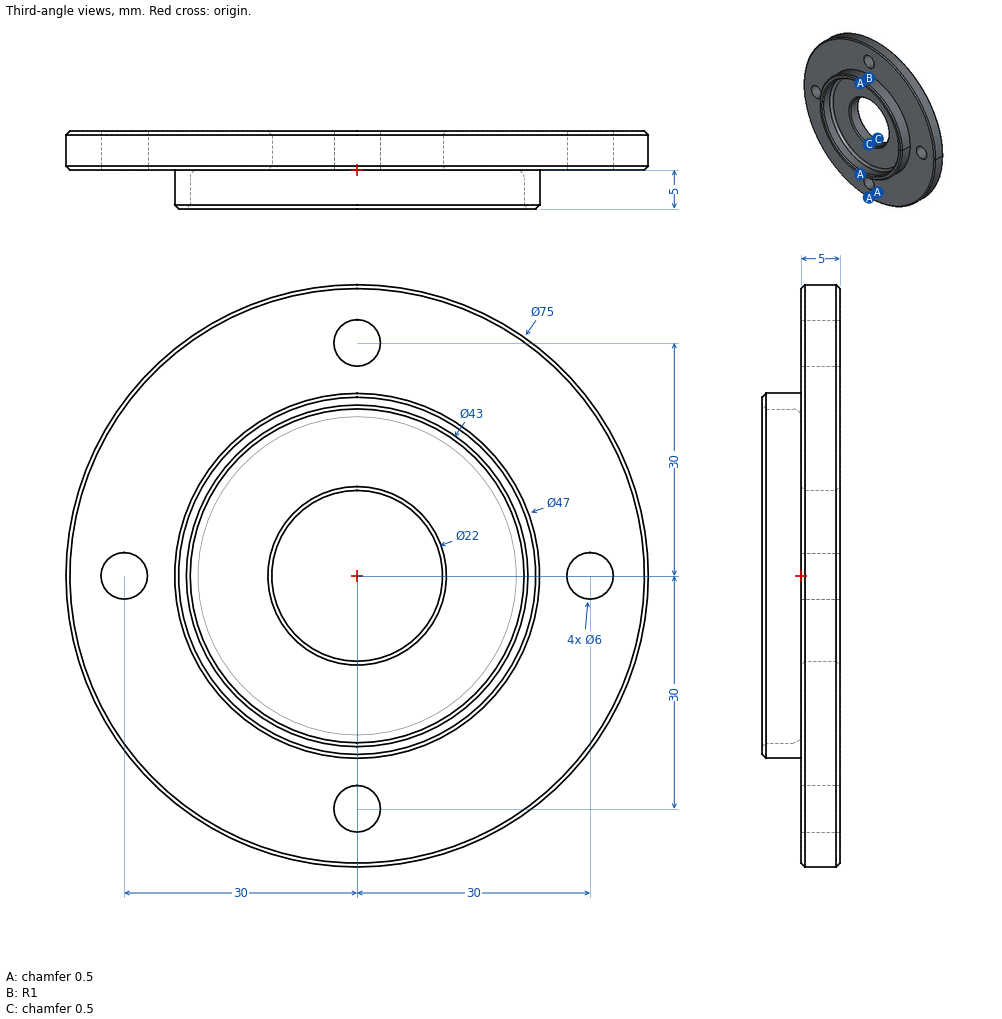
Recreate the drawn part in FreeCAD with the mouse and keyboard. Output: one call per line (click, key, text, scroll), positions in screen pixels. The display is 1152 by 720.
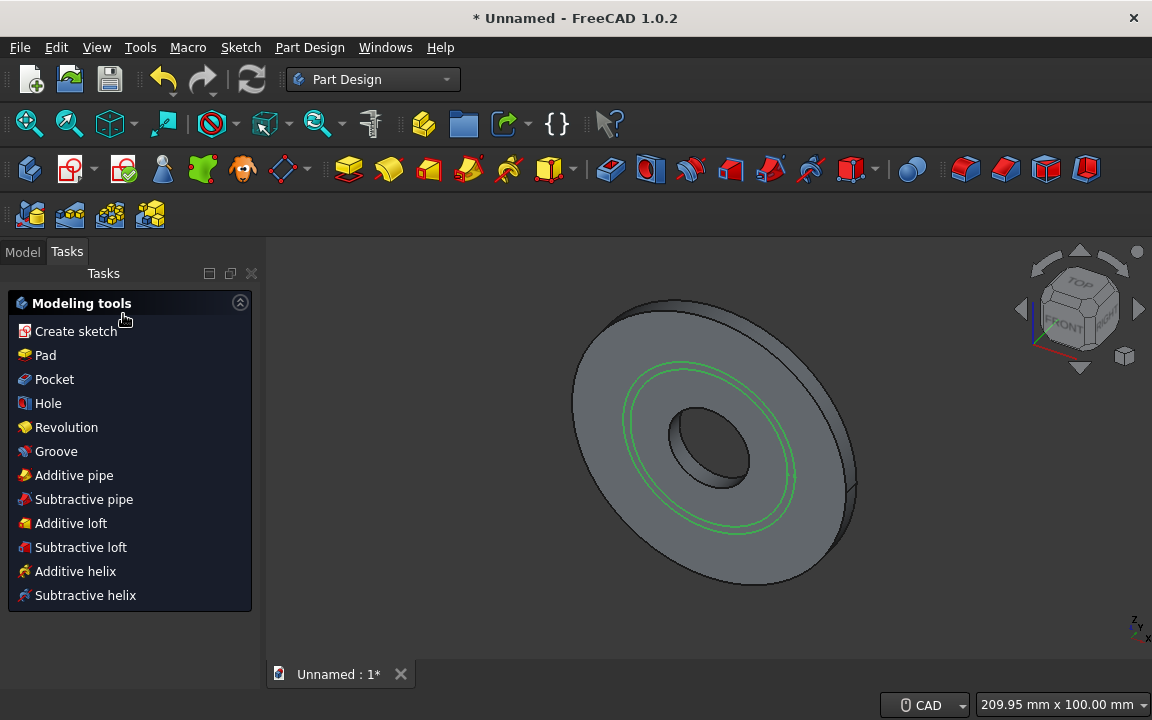
click(350, 170)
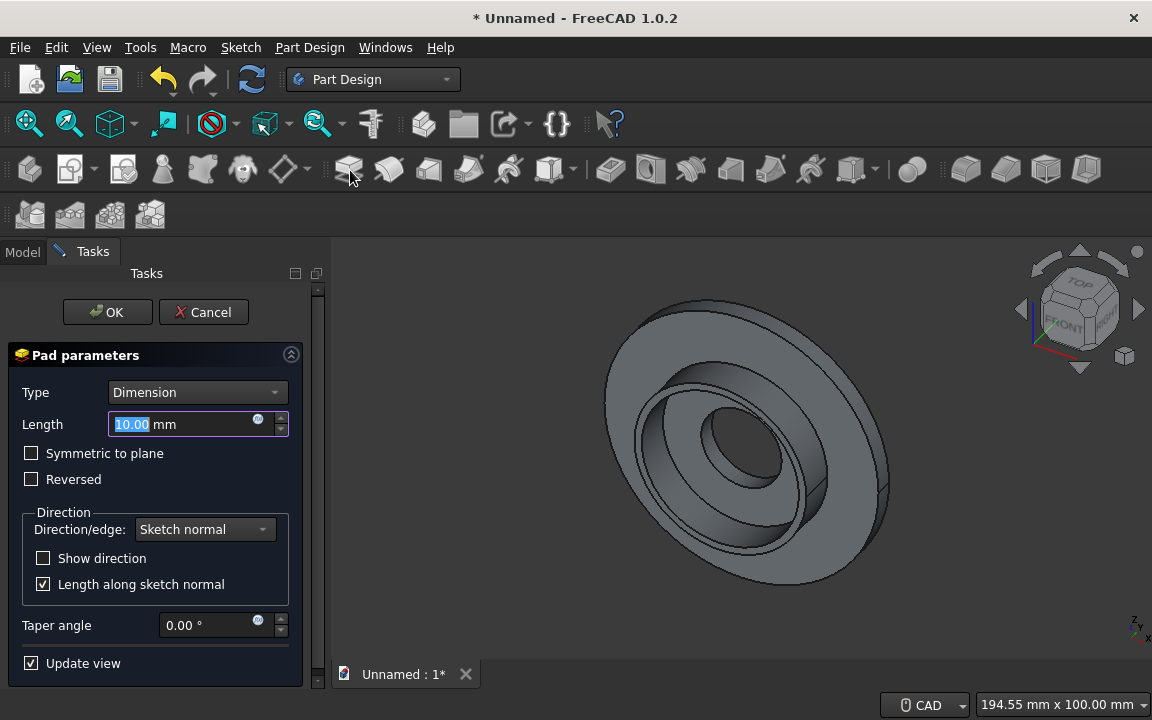
text(5)
key(Tab)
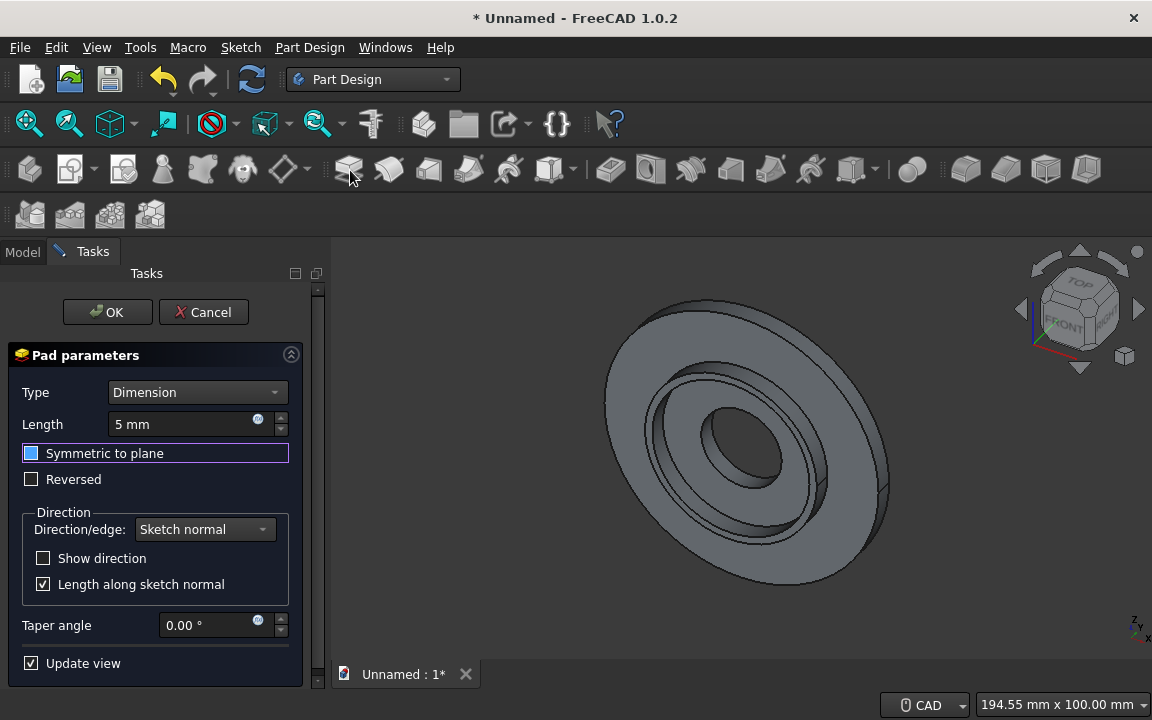
click(108, 312)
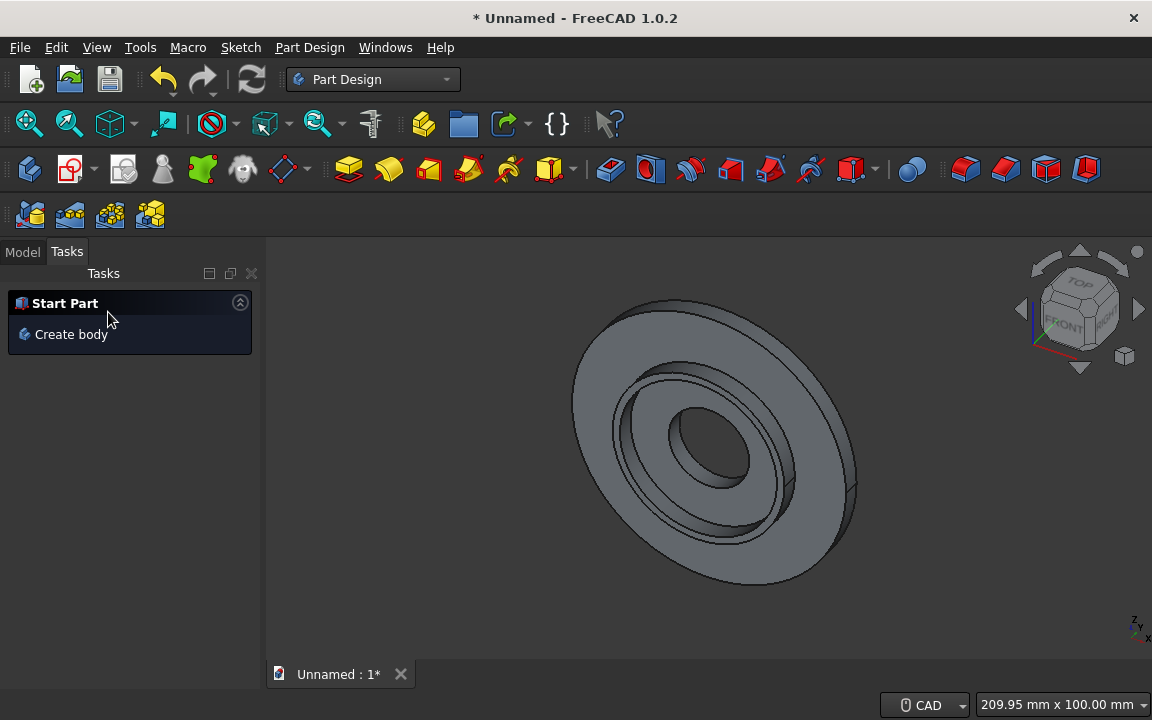
key(4)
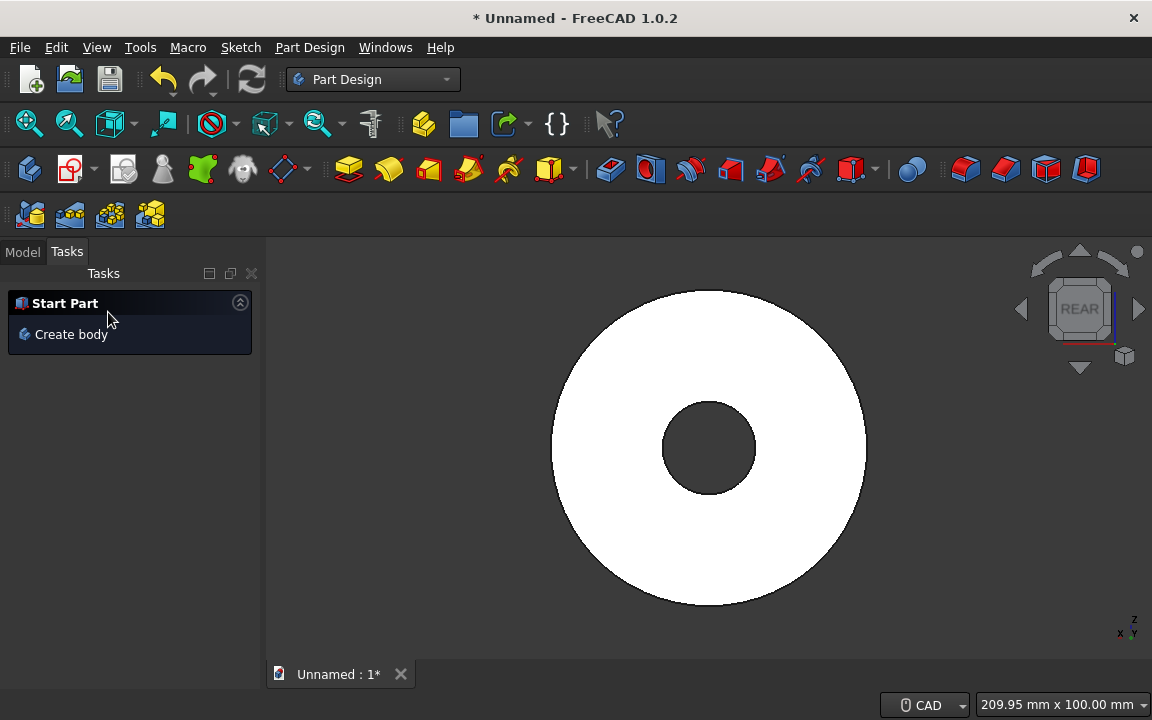
click(754, 357)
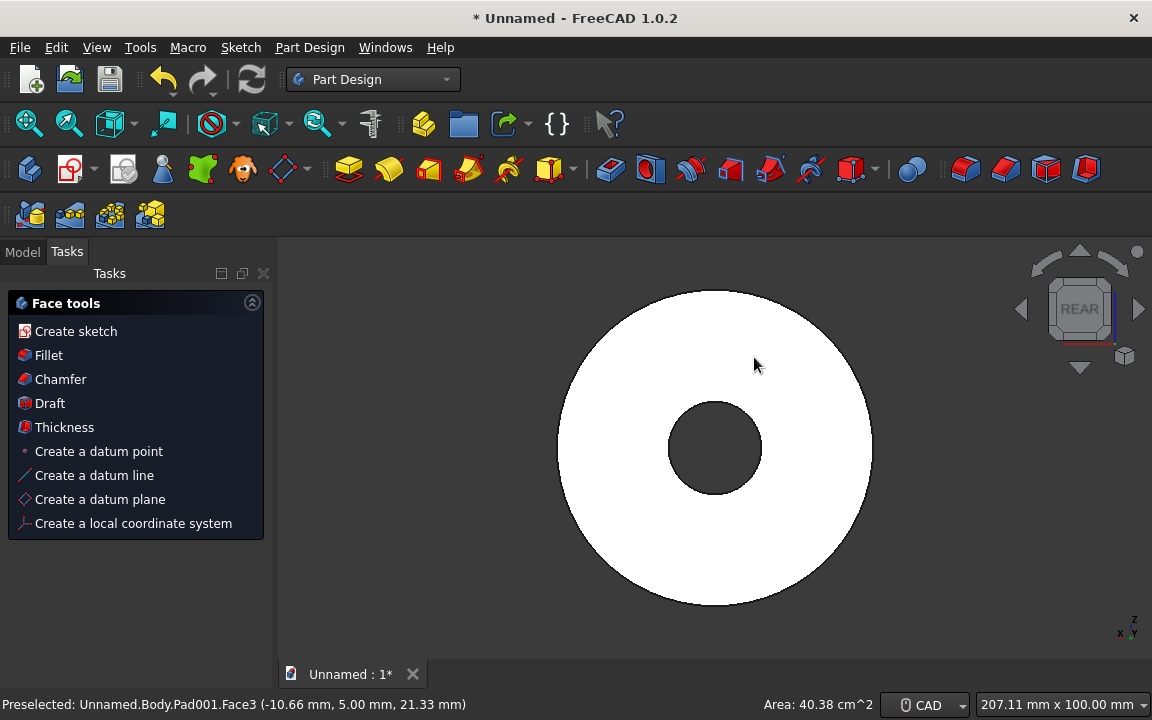
click(70, 170)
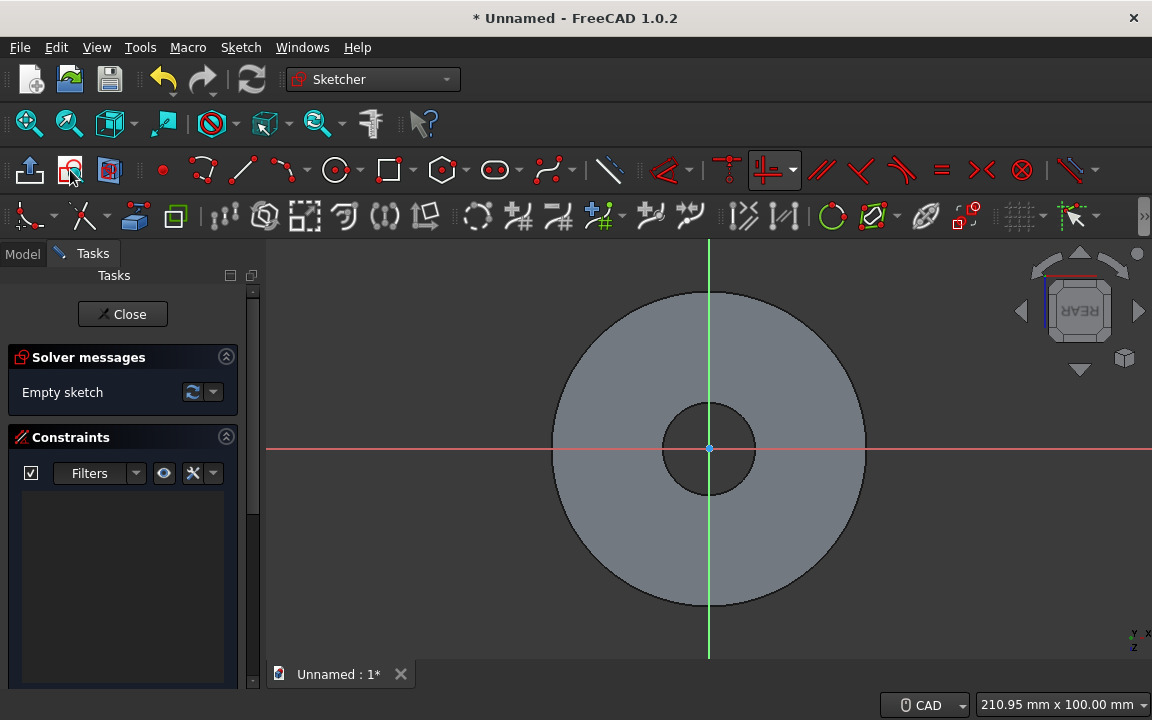
key(g)
key(c)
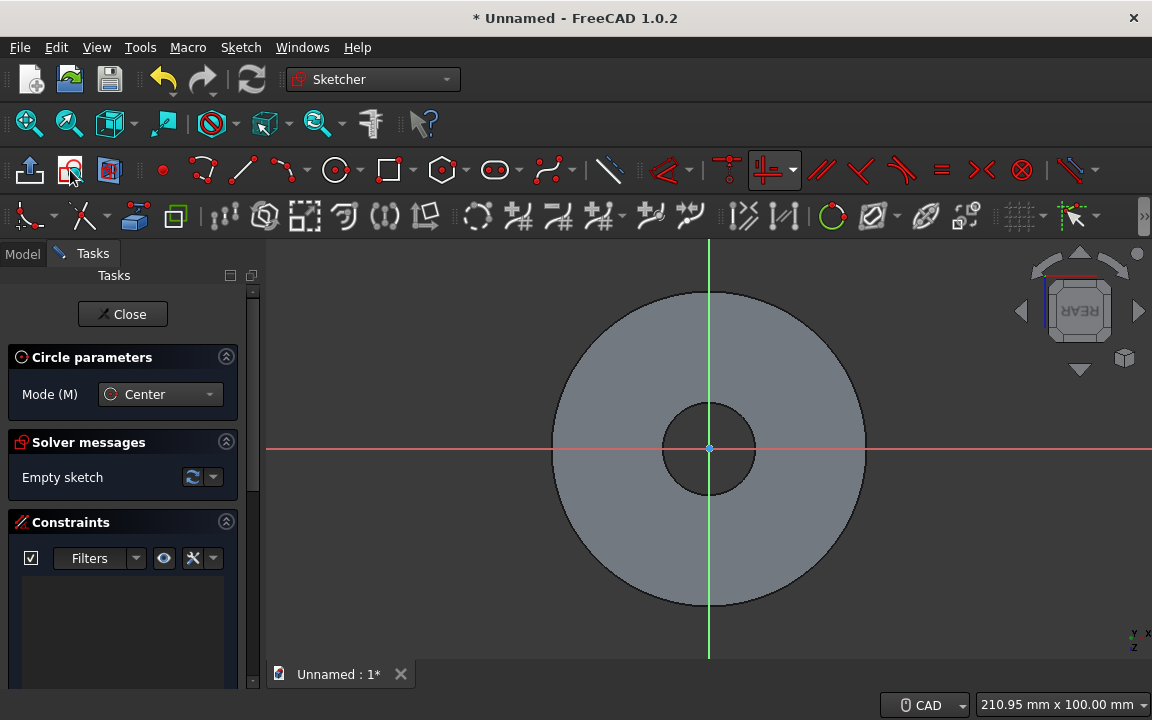
scroll(835, 449, up, 3)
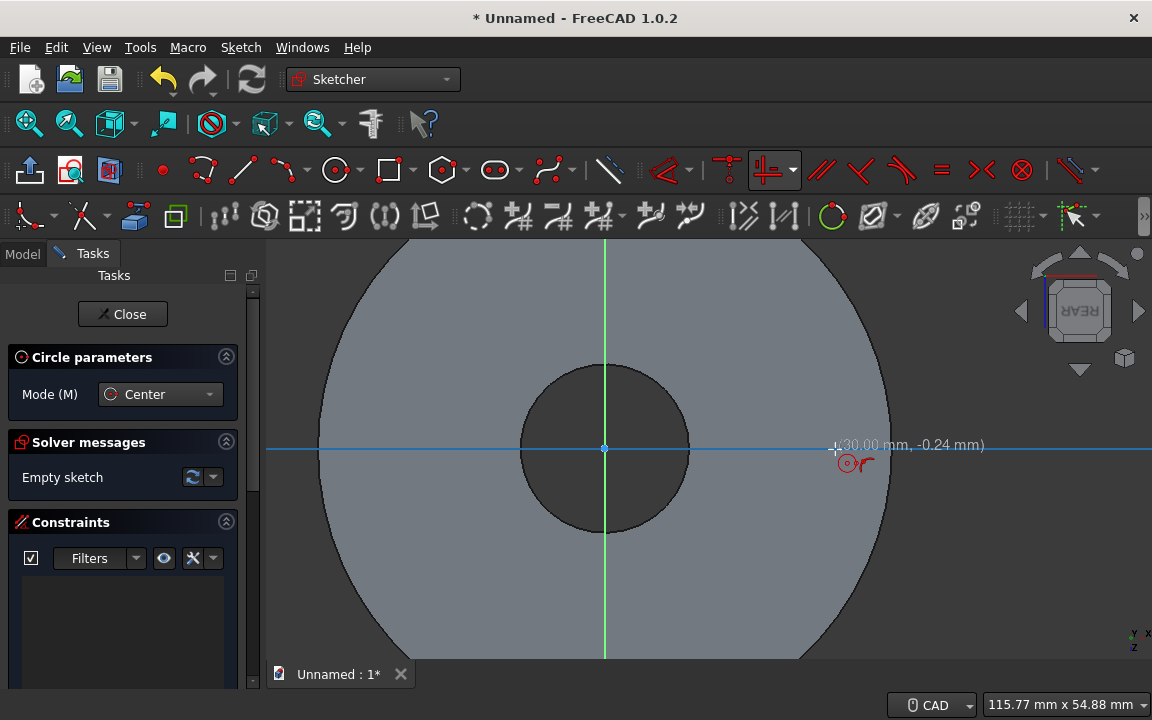
click(834, 449)
move(851, 432)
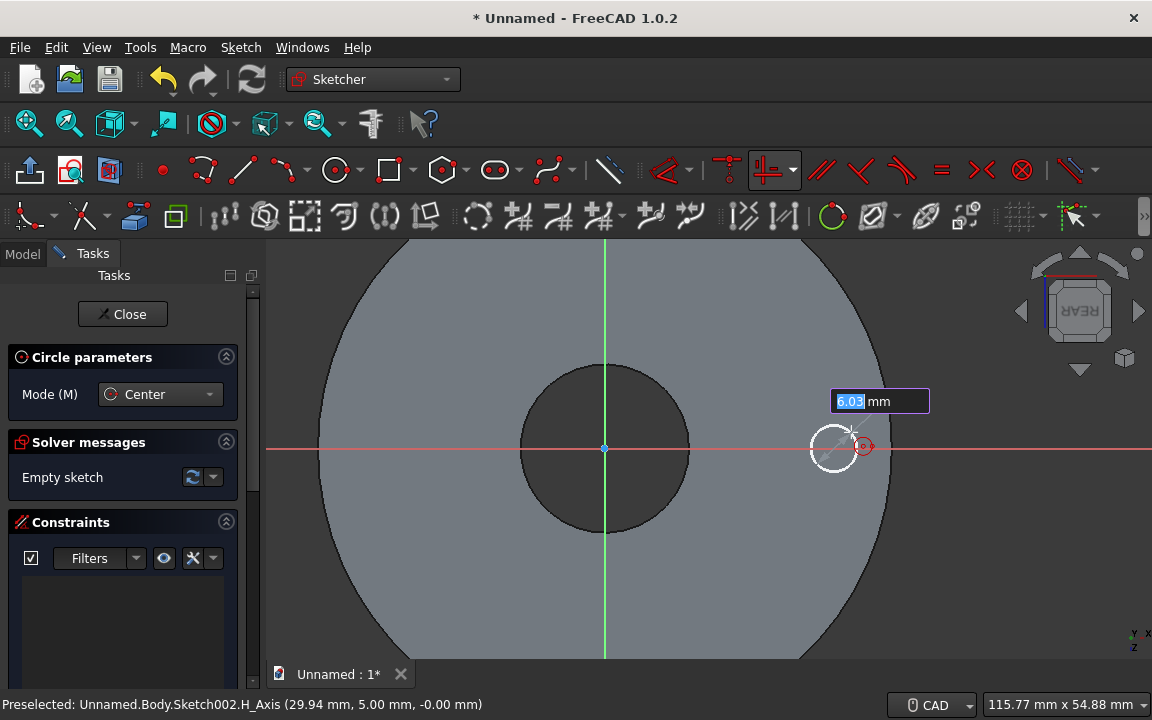
text(6)
key(Return)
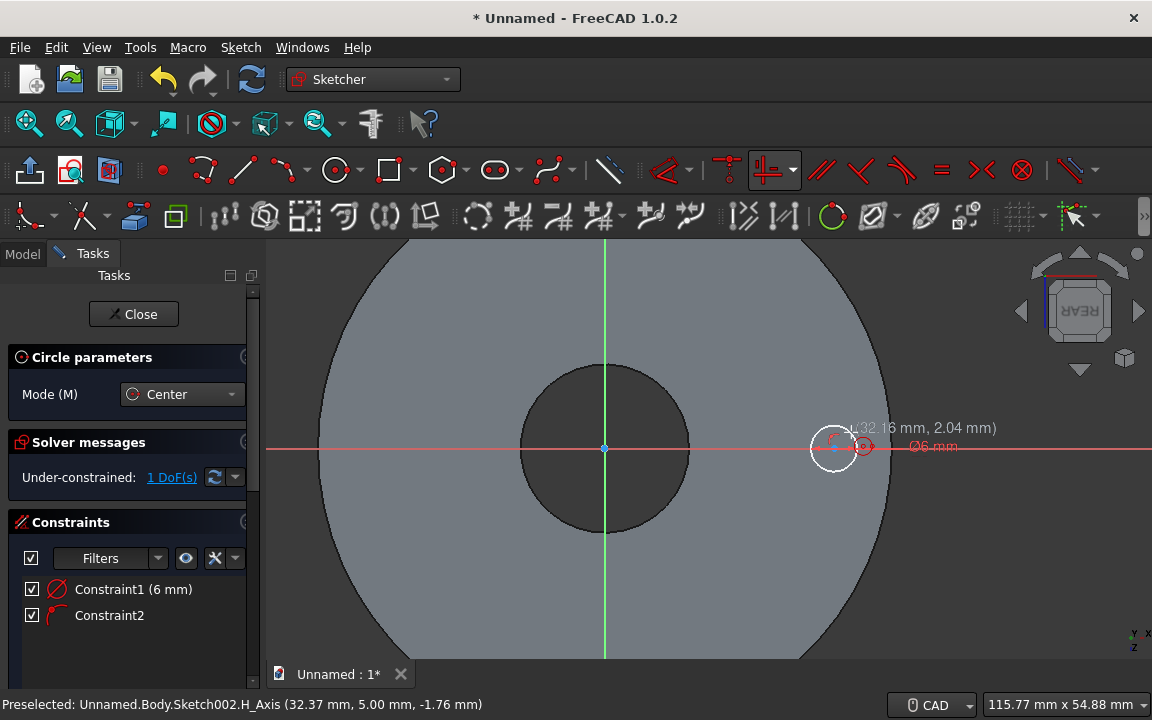
scroll(684, 450, down, 3)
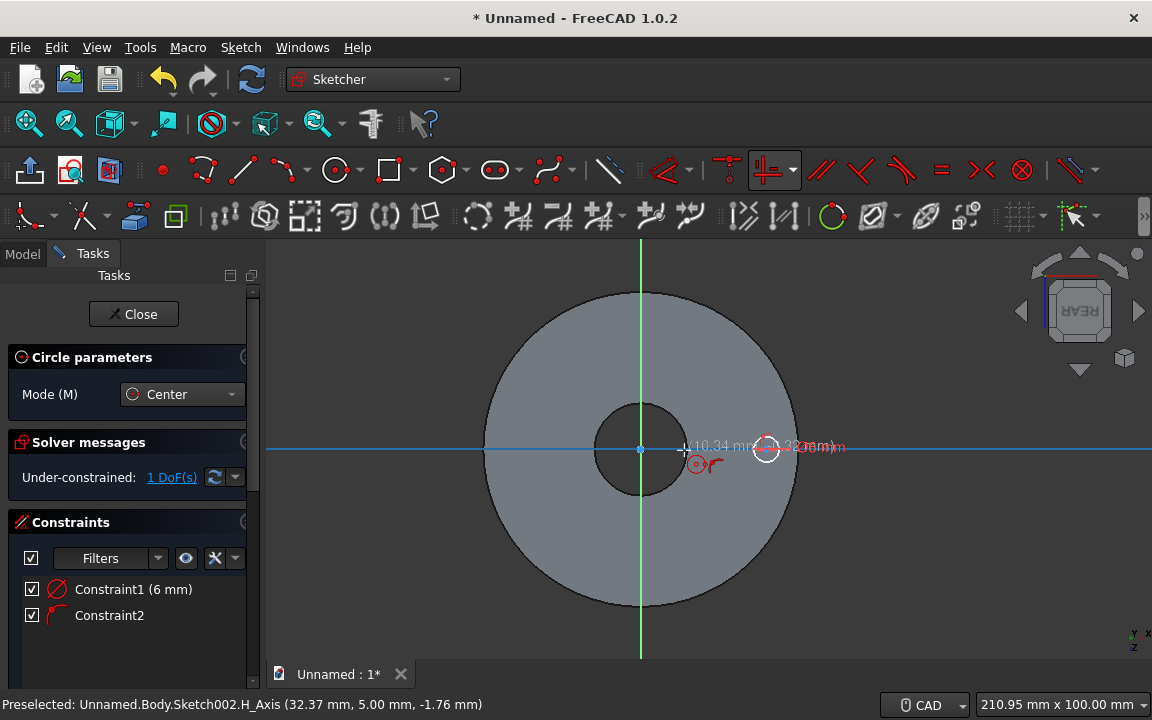
scroll(641, 575, up, 3)